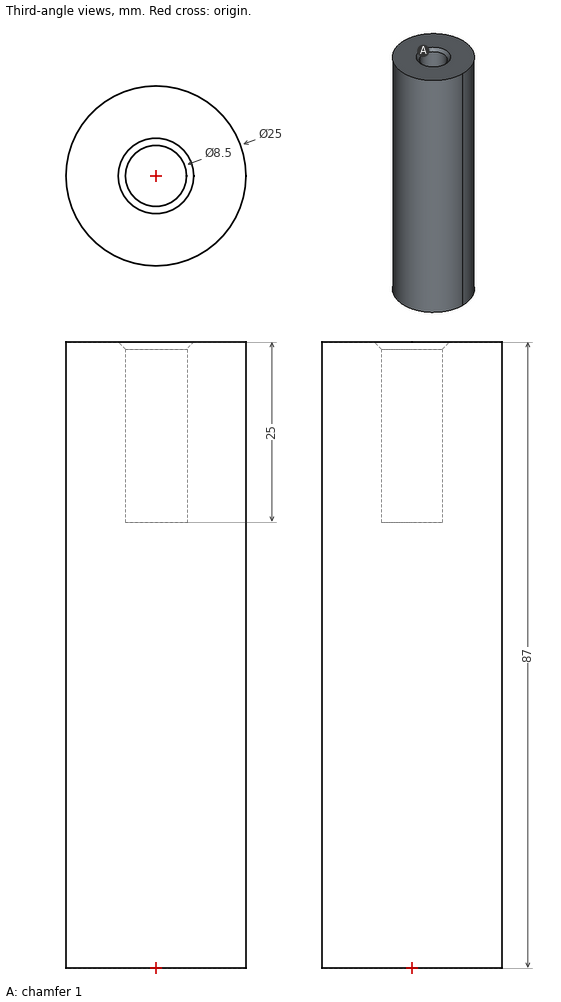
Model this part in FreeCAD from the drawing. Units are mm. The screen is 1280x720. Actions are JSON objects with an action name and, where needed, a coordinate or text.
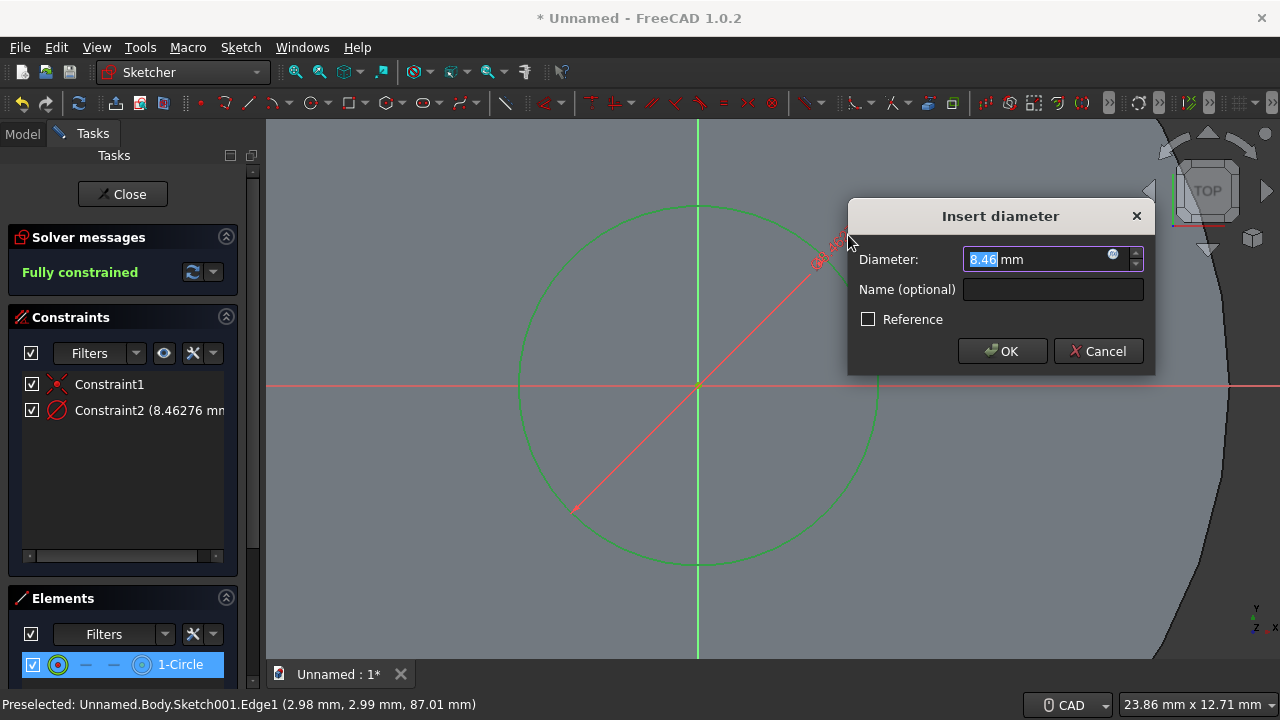
{"action": "type", "text": "8.5"}
{"action": "key", "text": "Return"}
{"action": "key", "text": "Escape"}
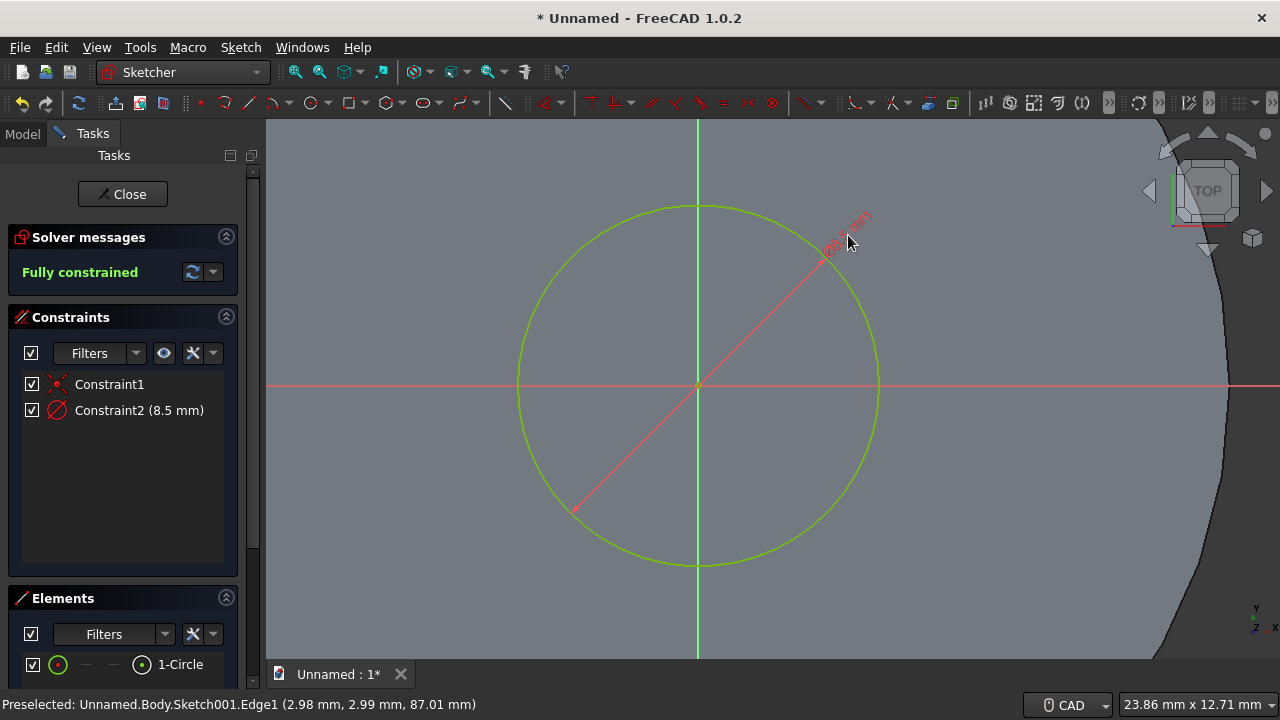
{"action": "left_click", "coordinate": [123, 194]}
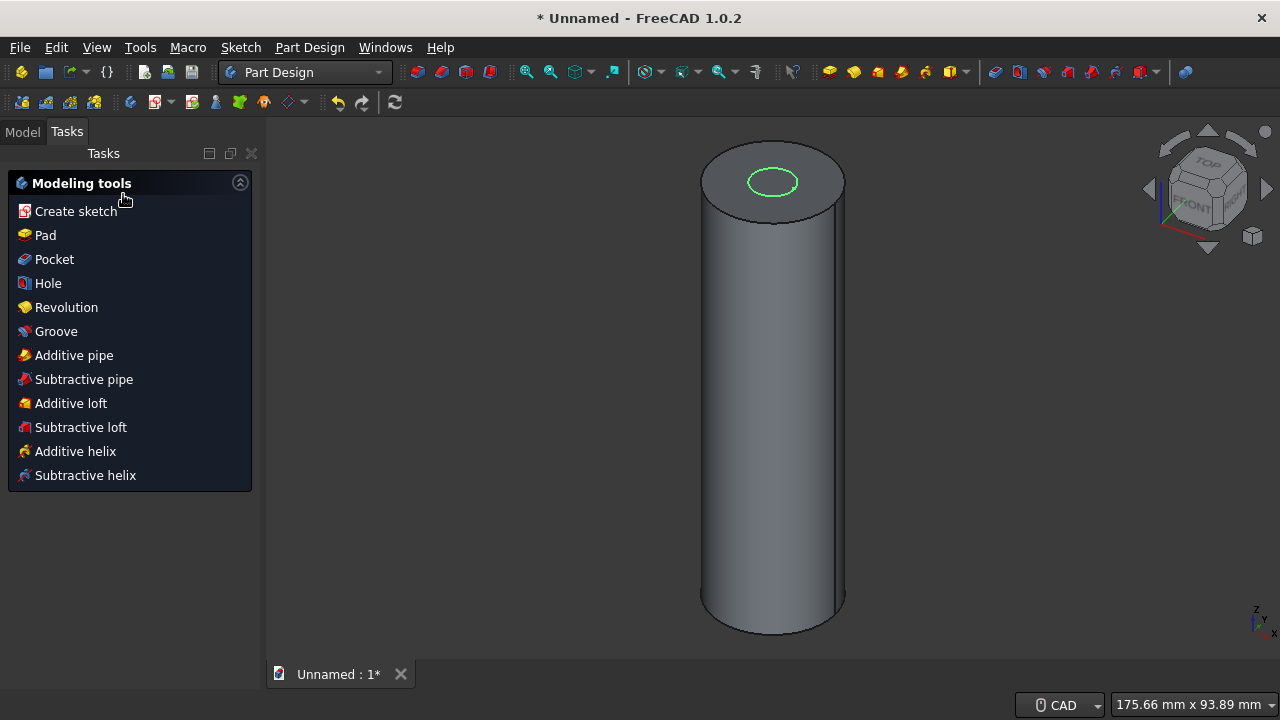
{"action": "left_click", "coordinate": [996, 72]}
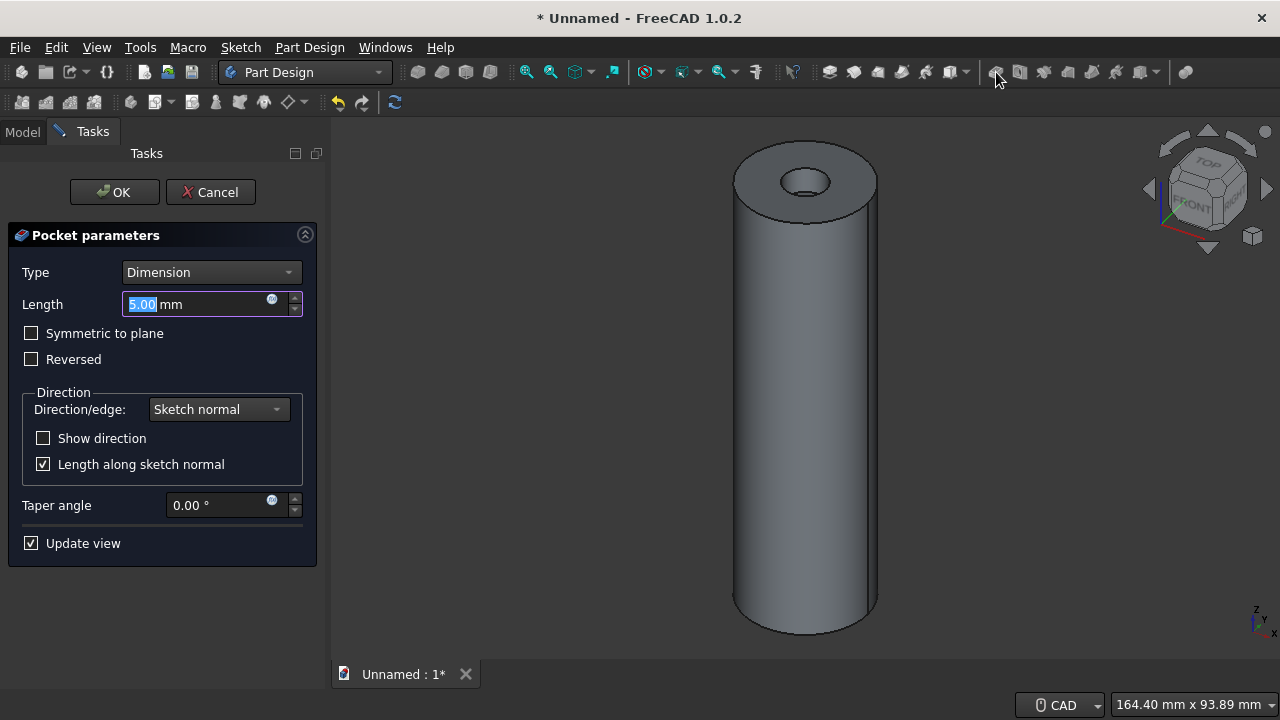
{"action": "type", "text": "25"}
{"action": "key", "text": "Tab"}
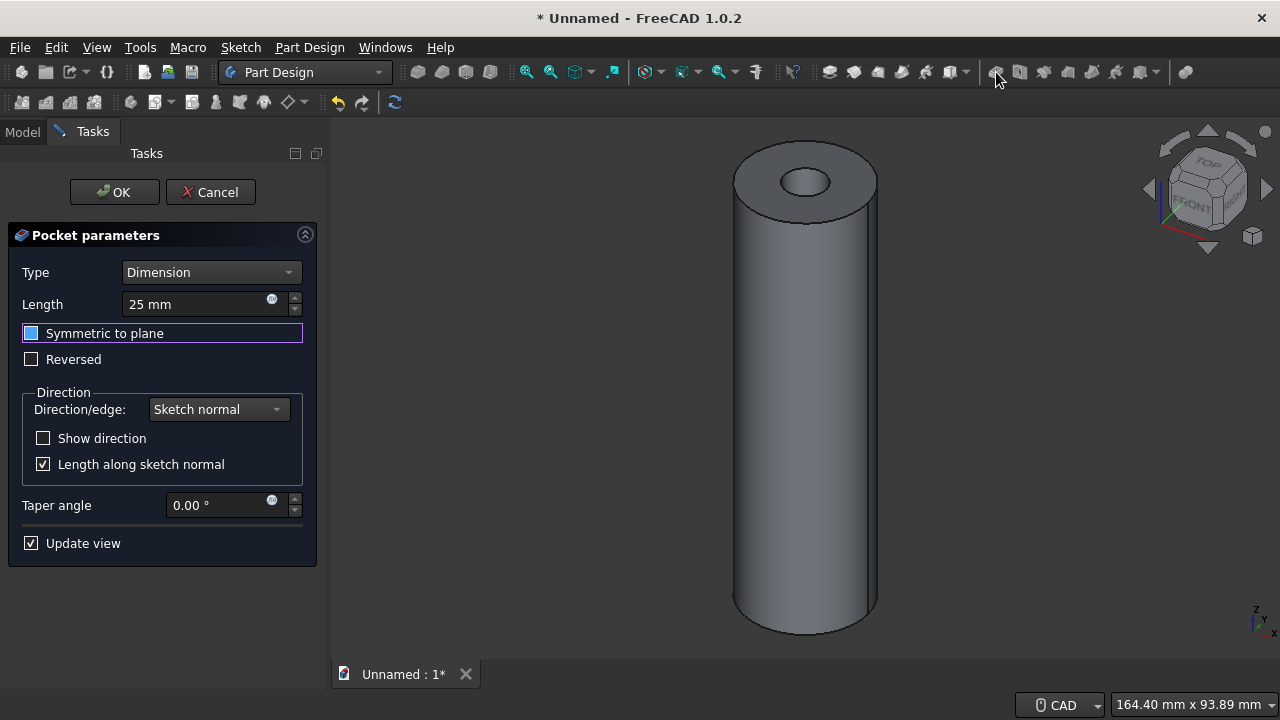
{"action": "left_click", "coordinate": [115, 192]}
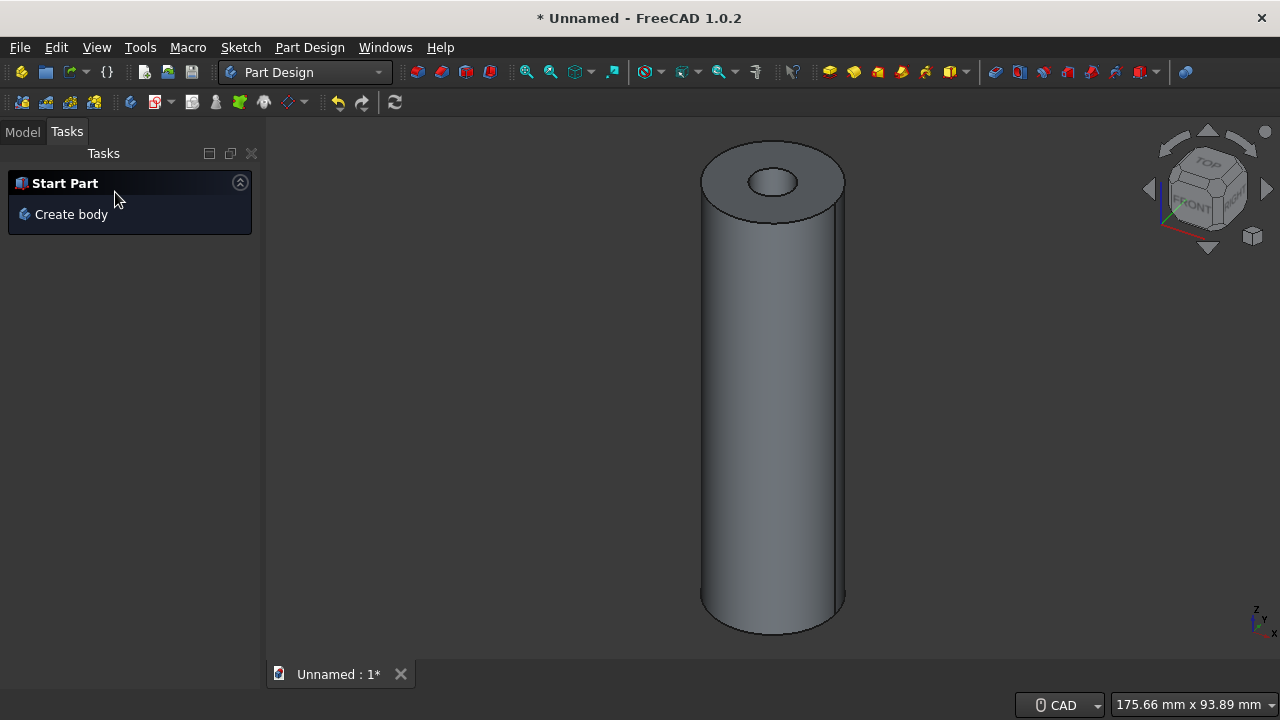
{"action": "left_click", "coordinate": [752, 174]}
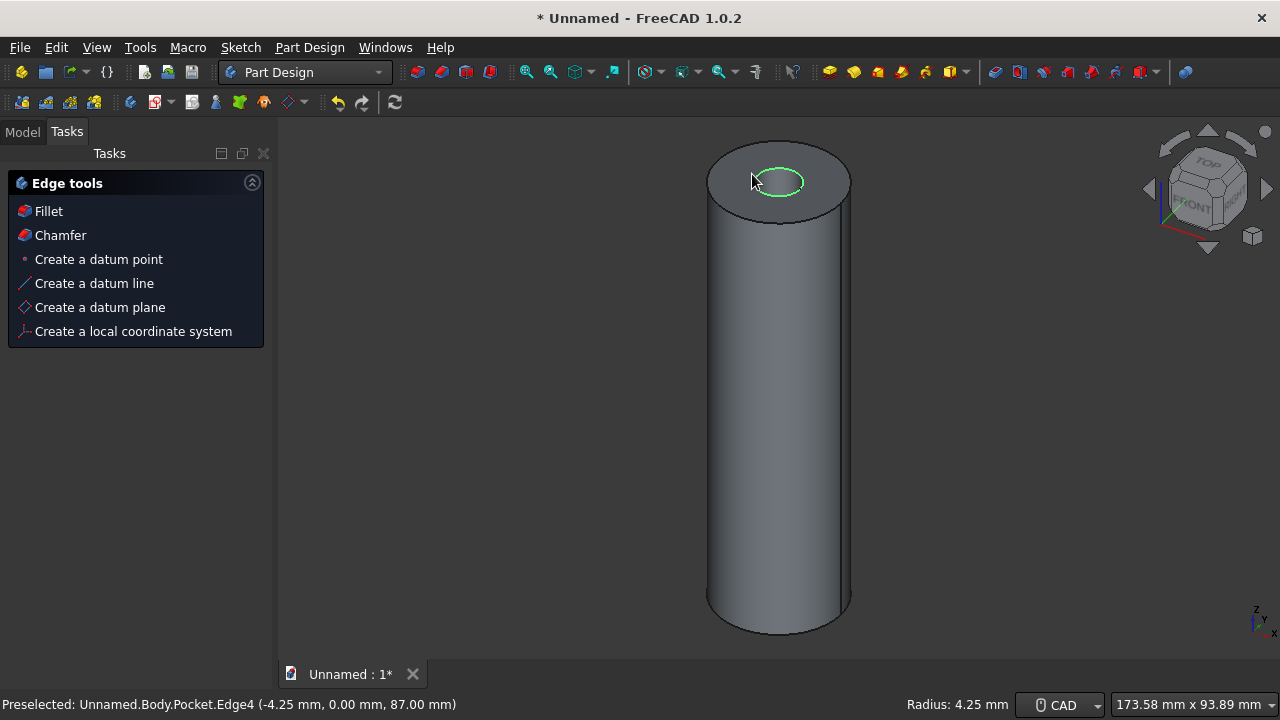
{"action": "left_click", "coordinate": [442, 72]}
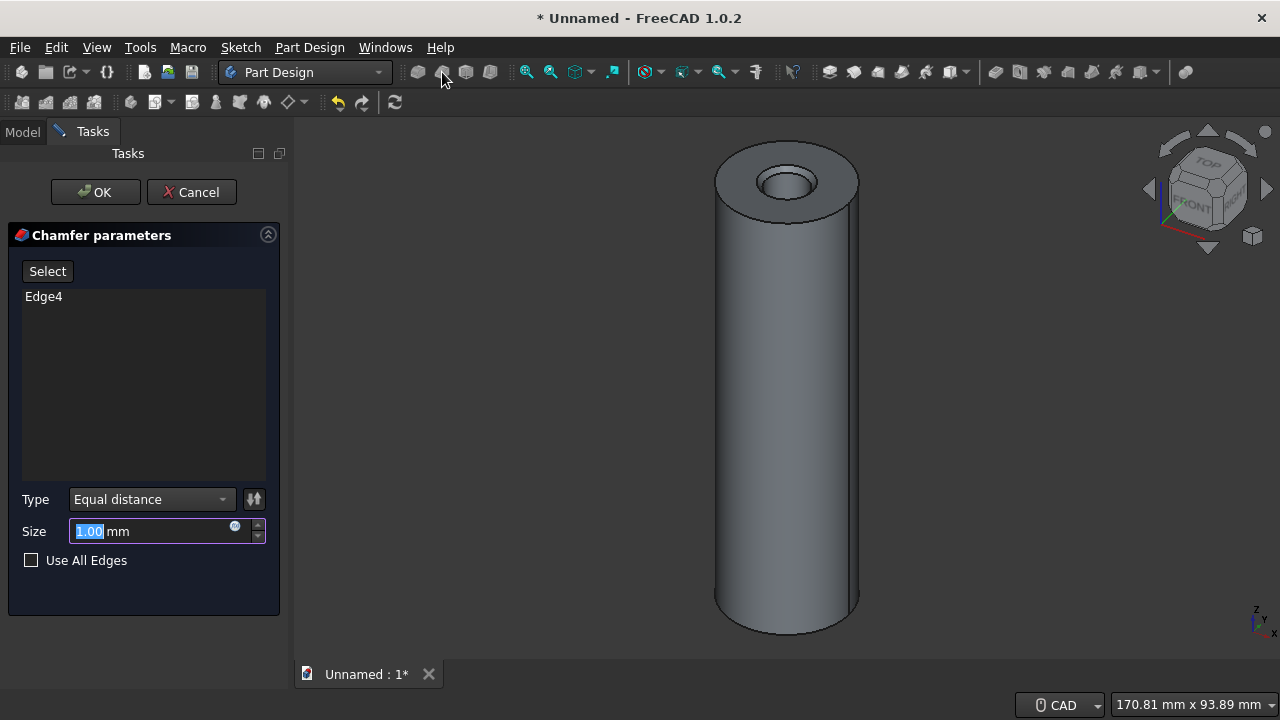
{"action": "type", "text": "1"}
{"action": "key", "text": "Tab"}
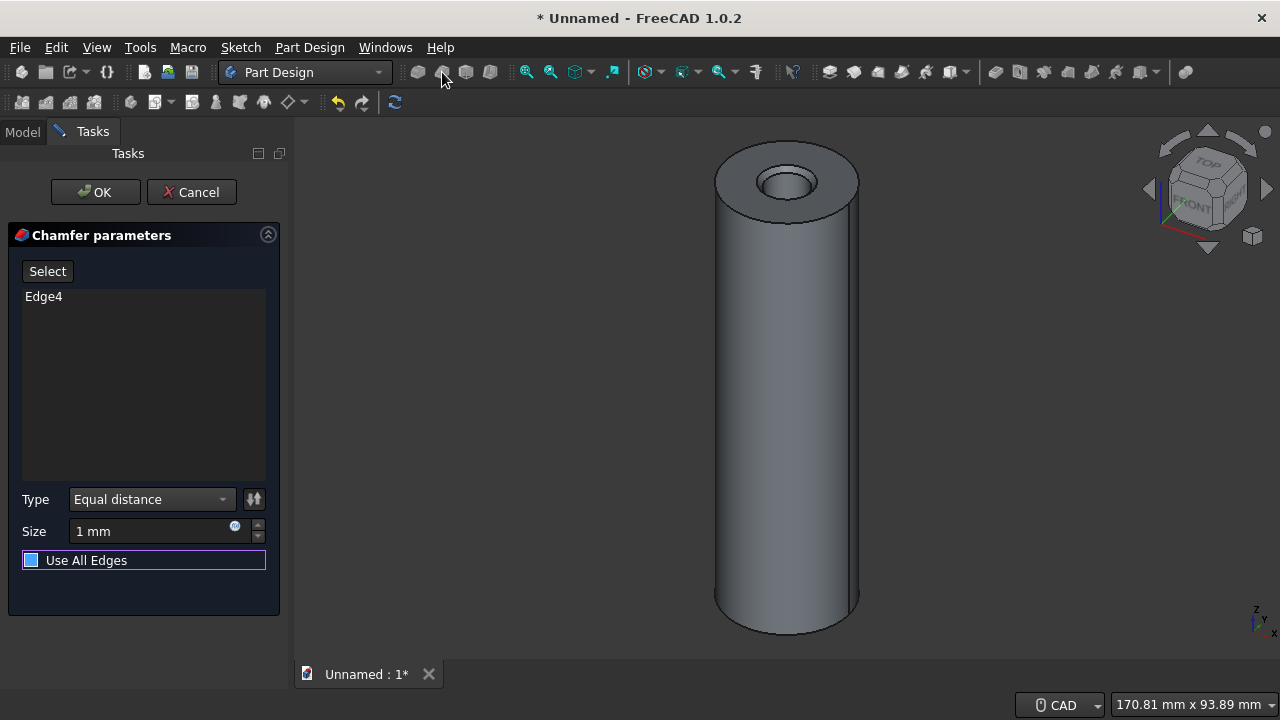
{"action": "left_click", "coordinate": [96, 192]}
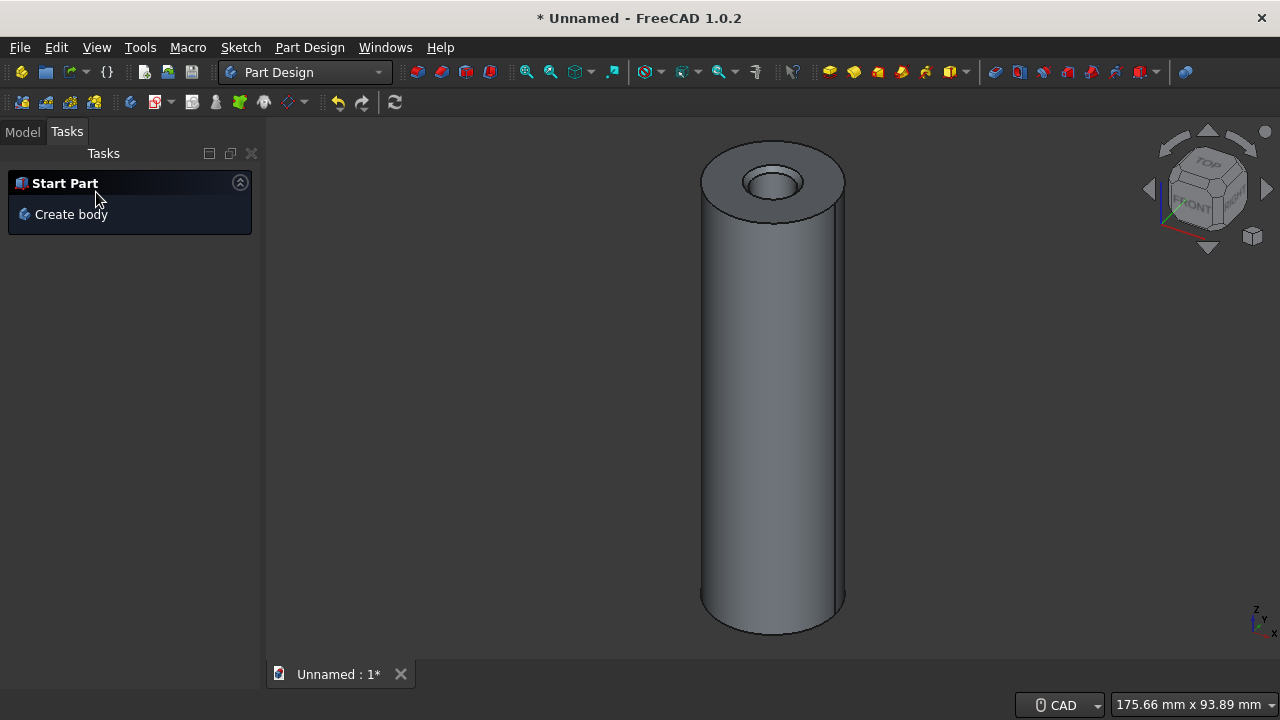
{"action": "key", "text": "0"}